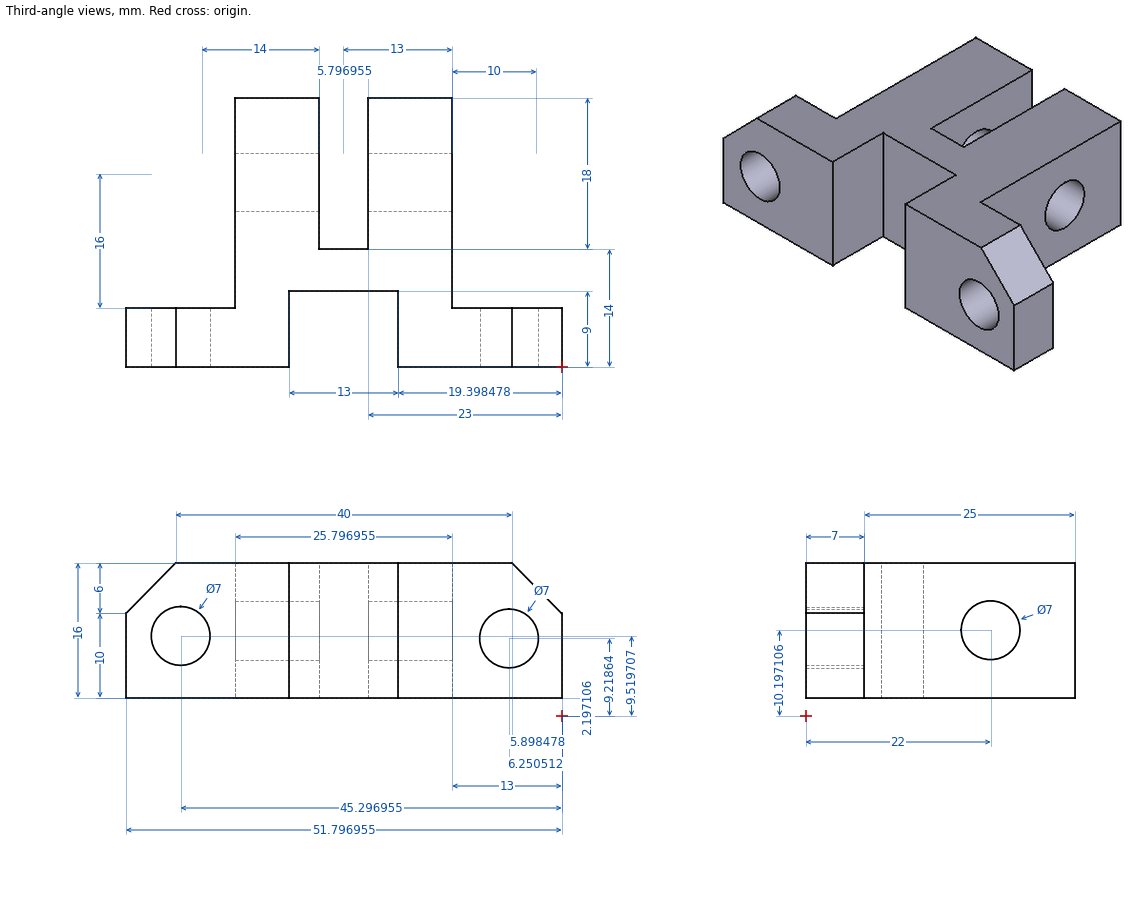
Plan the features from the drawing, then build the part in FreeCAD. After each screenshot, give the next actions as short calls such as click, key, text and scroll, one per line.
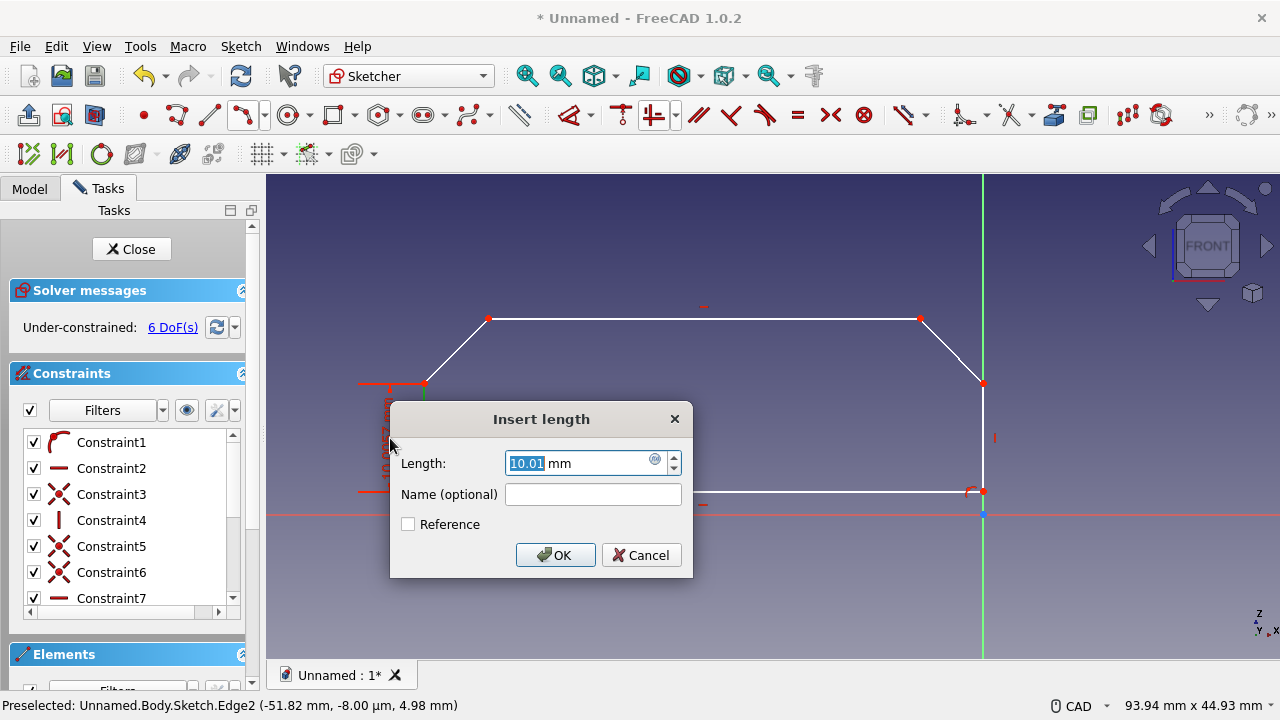
text(10)
key(Return)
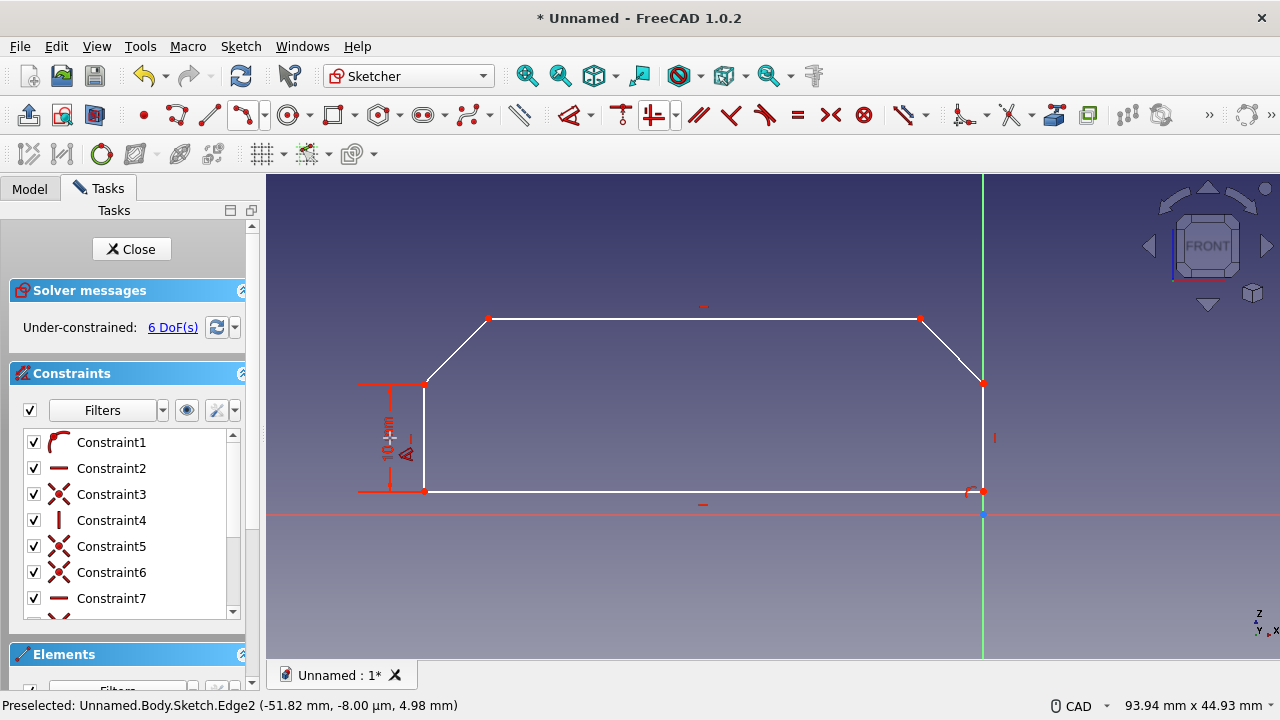
click(618, 319)
click(704, 285)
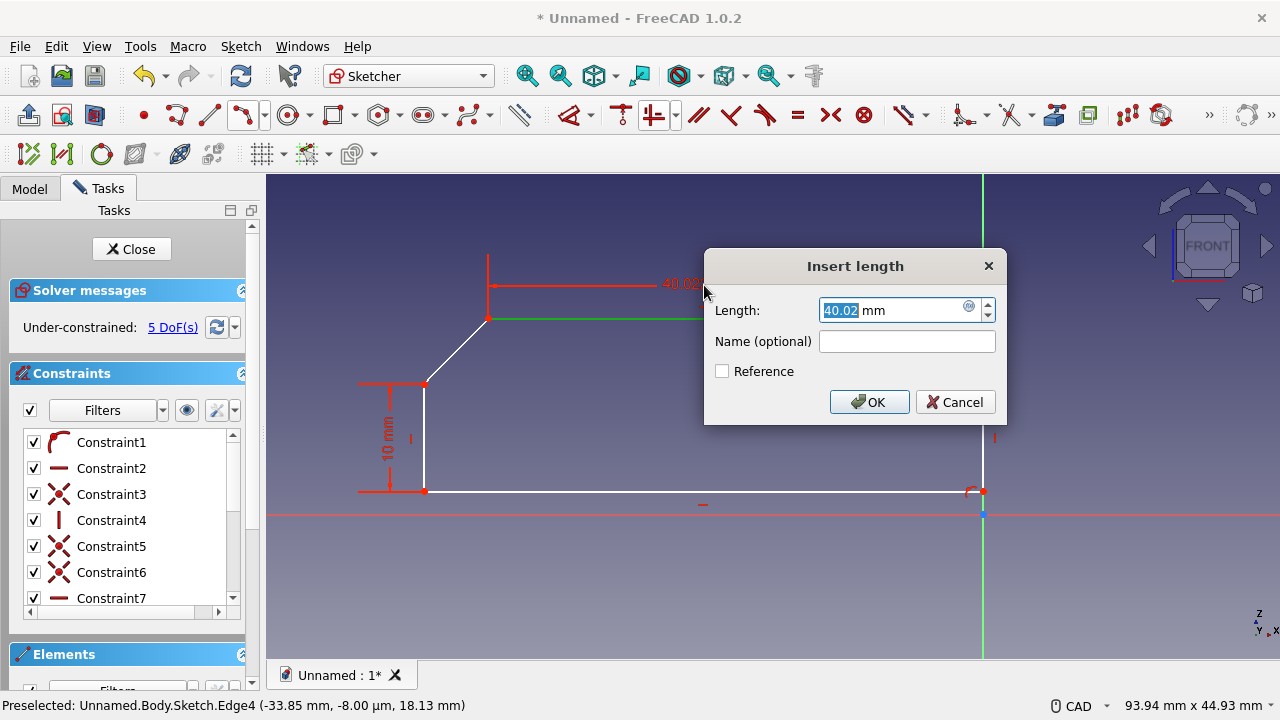
text(40)
key(Return)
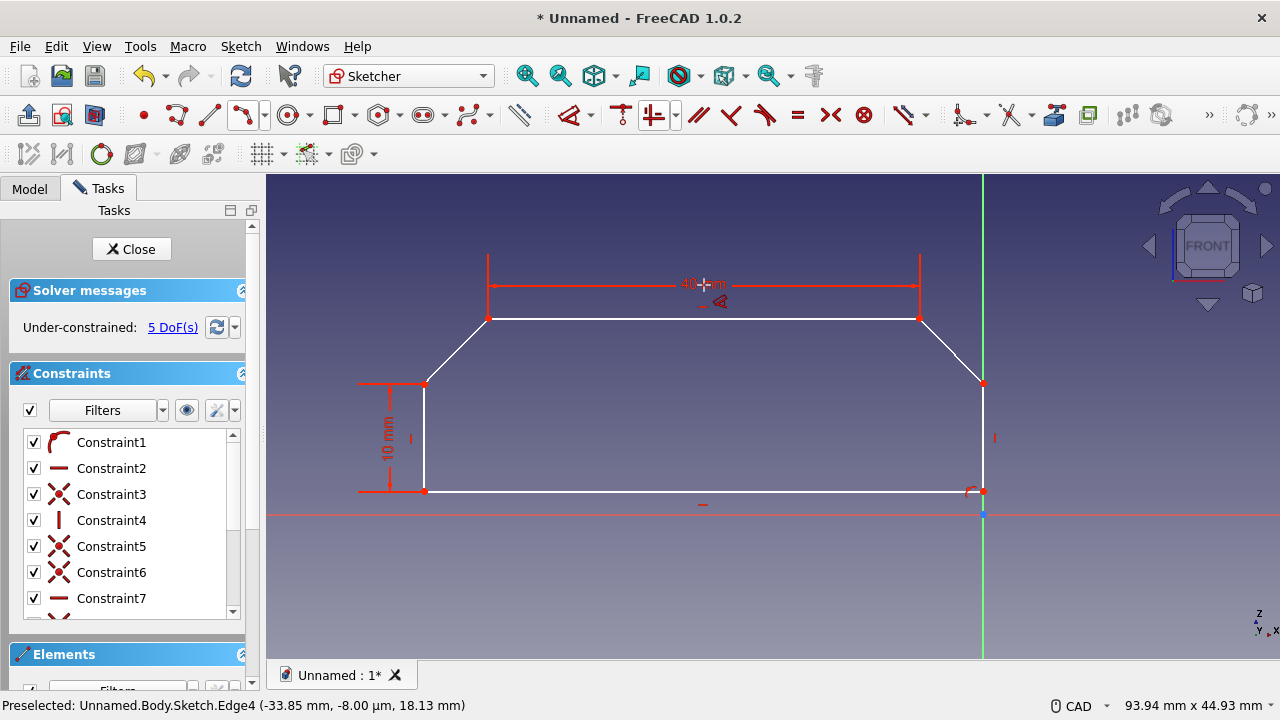
click(983, 416)
click(1017, 438)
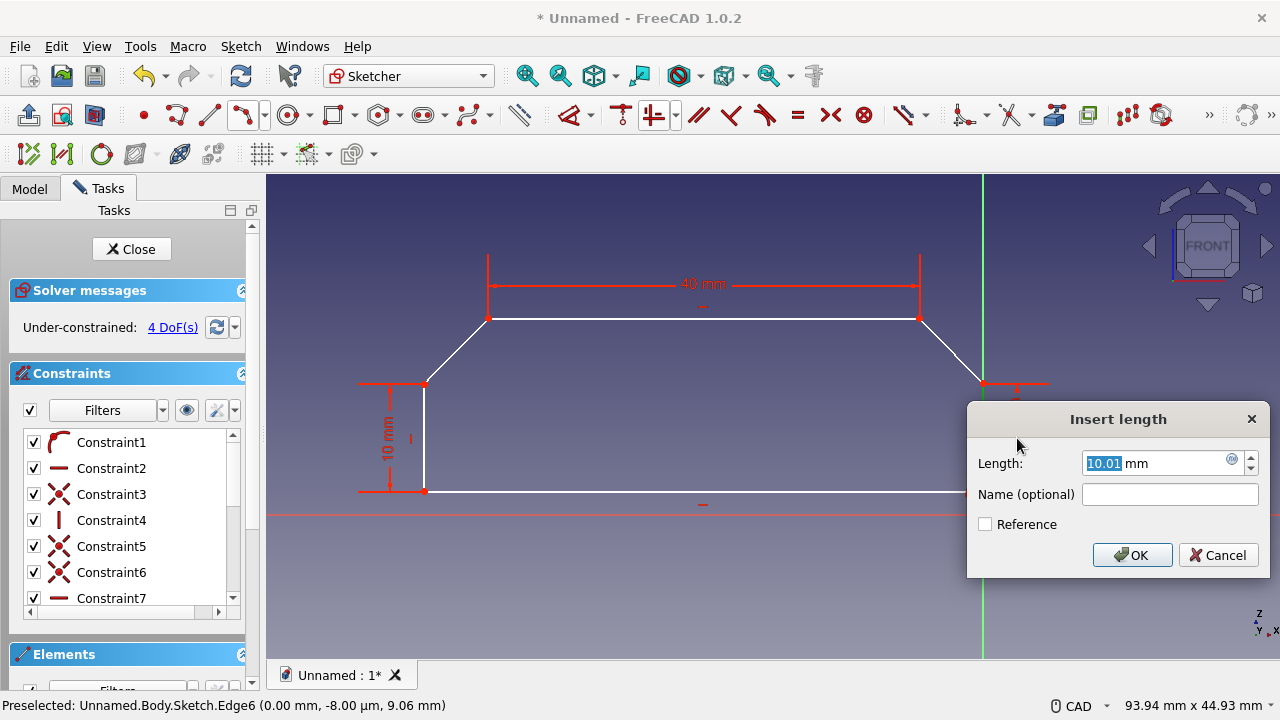
text(10)
key(Return)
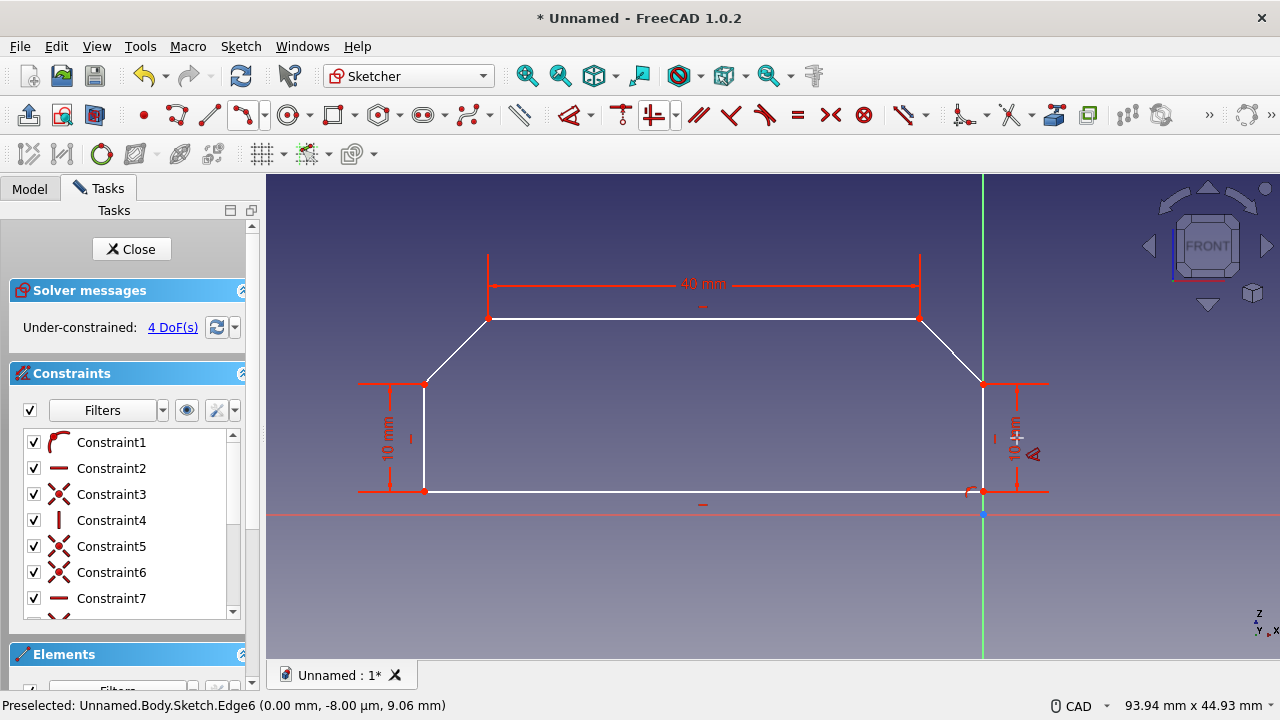
click(443, 365)
click(390, 352)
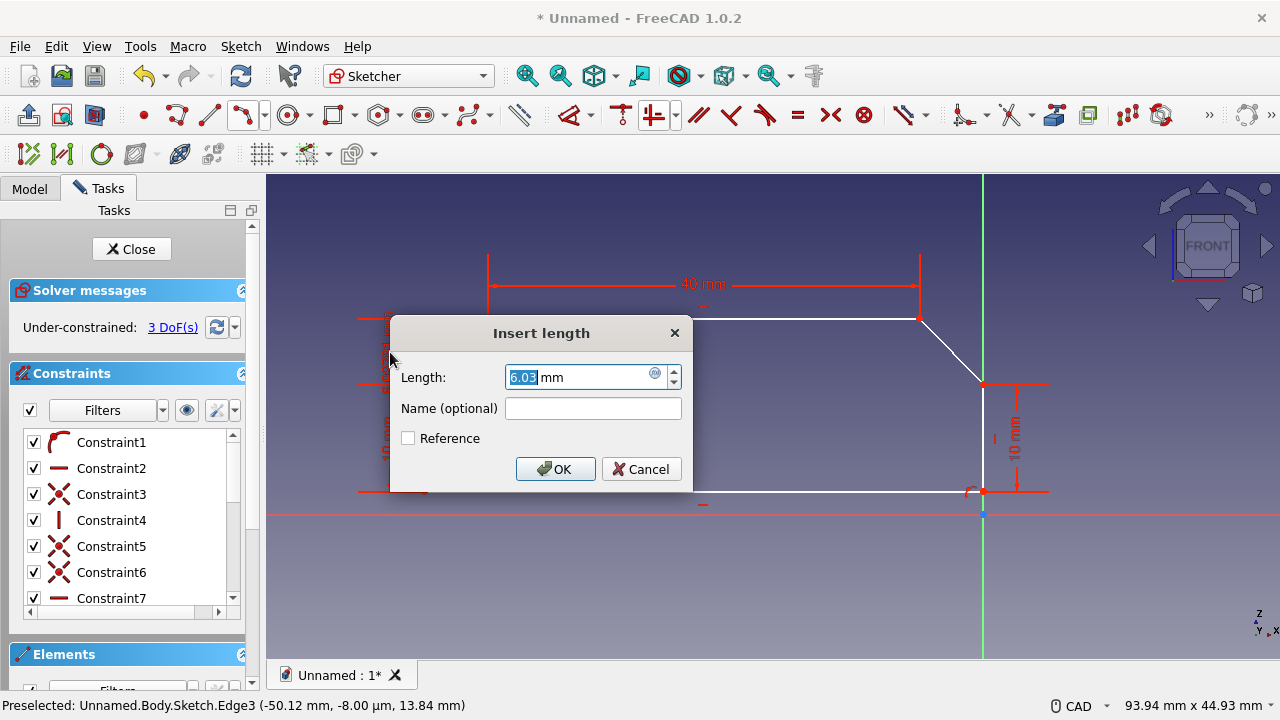
text(6)
key(Return)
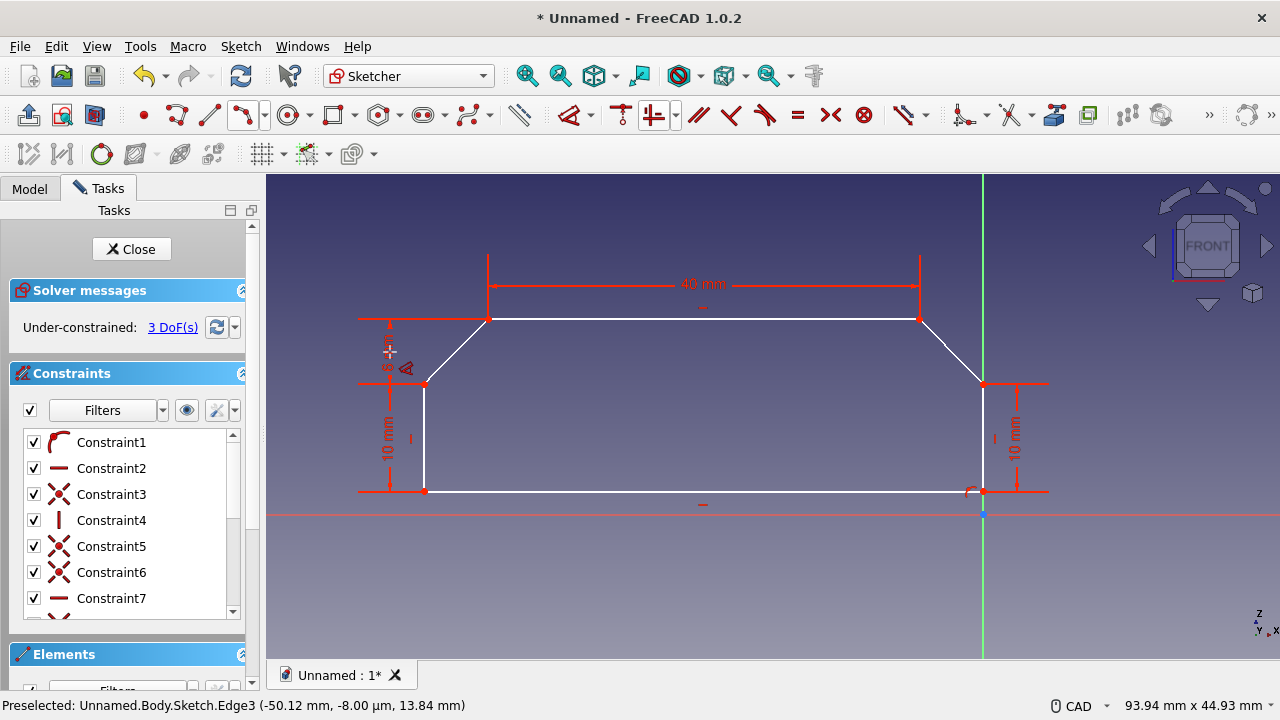
click(816, 492)
click(704, 458)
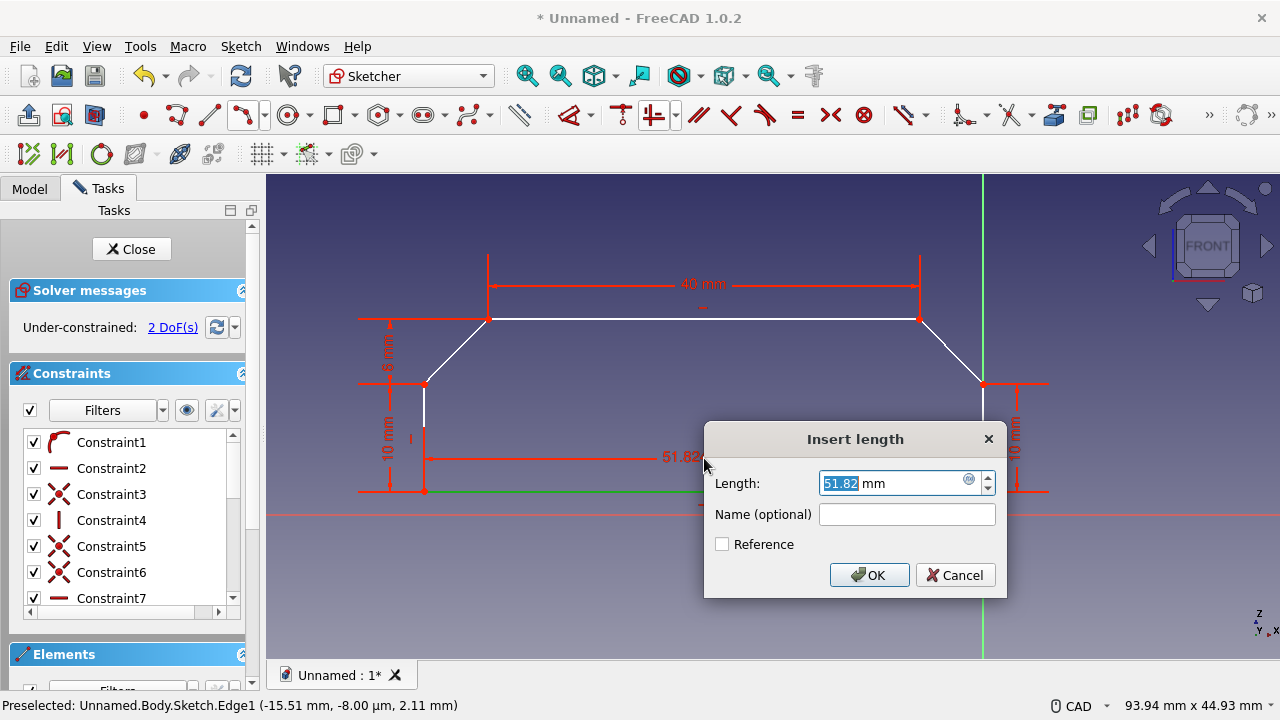
text(51.796955)
key(Return)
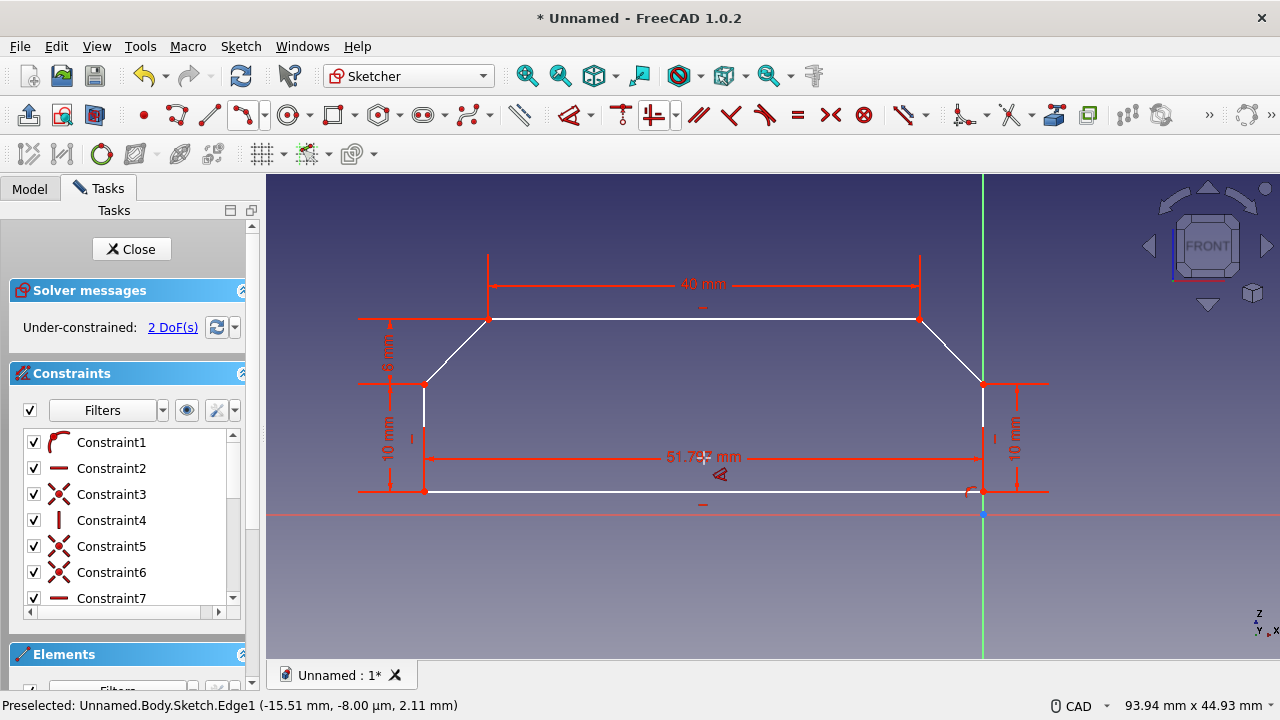
scroll(983, 492, up, 3)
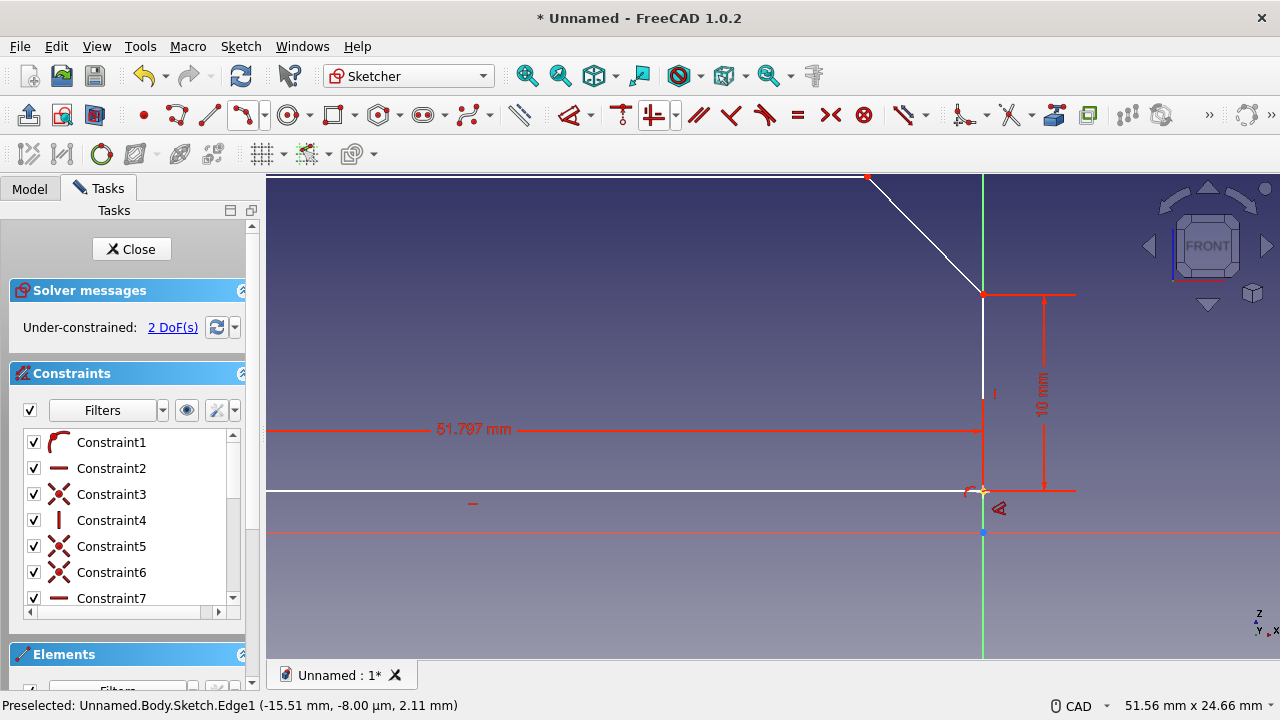
click(983, 491)
click(1017, 512)